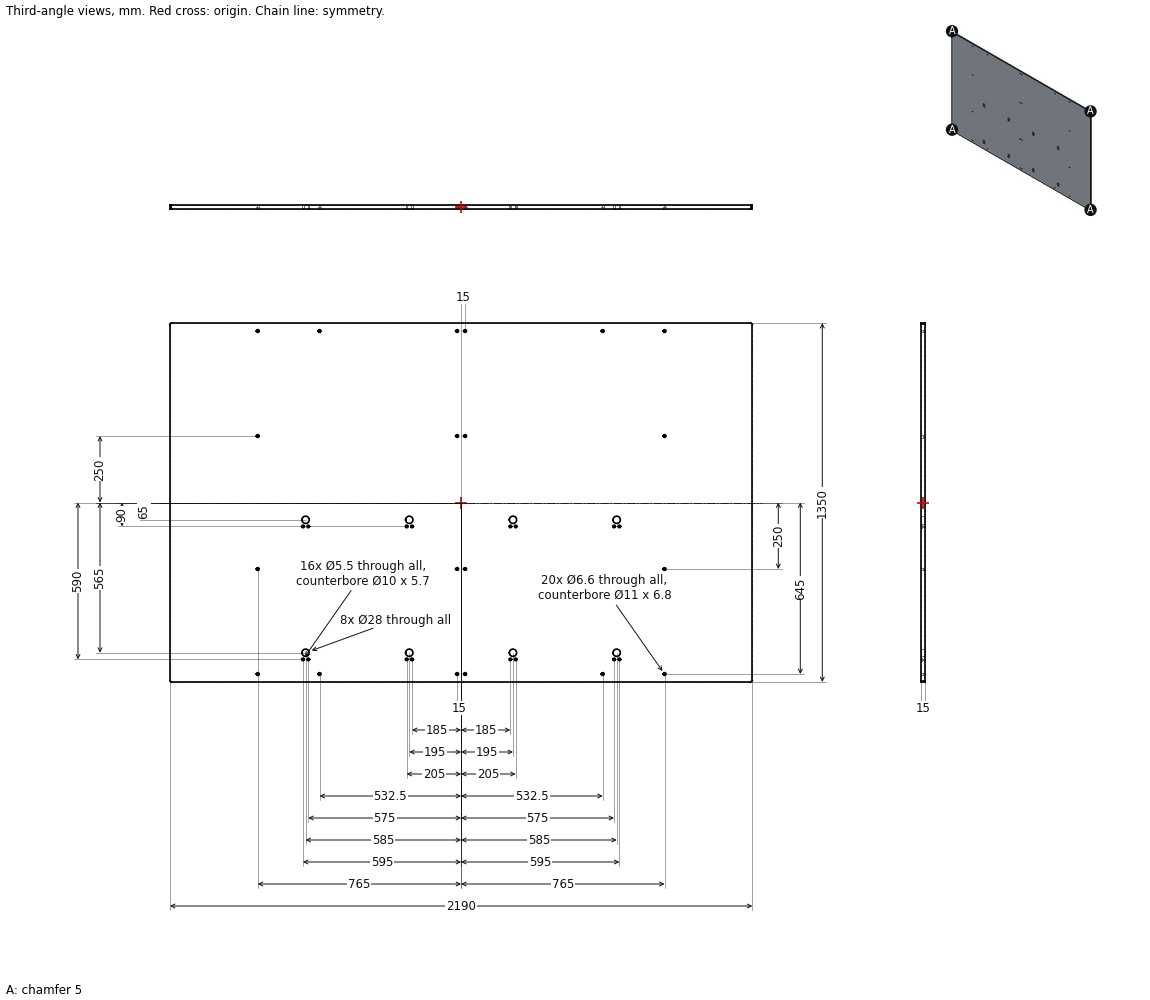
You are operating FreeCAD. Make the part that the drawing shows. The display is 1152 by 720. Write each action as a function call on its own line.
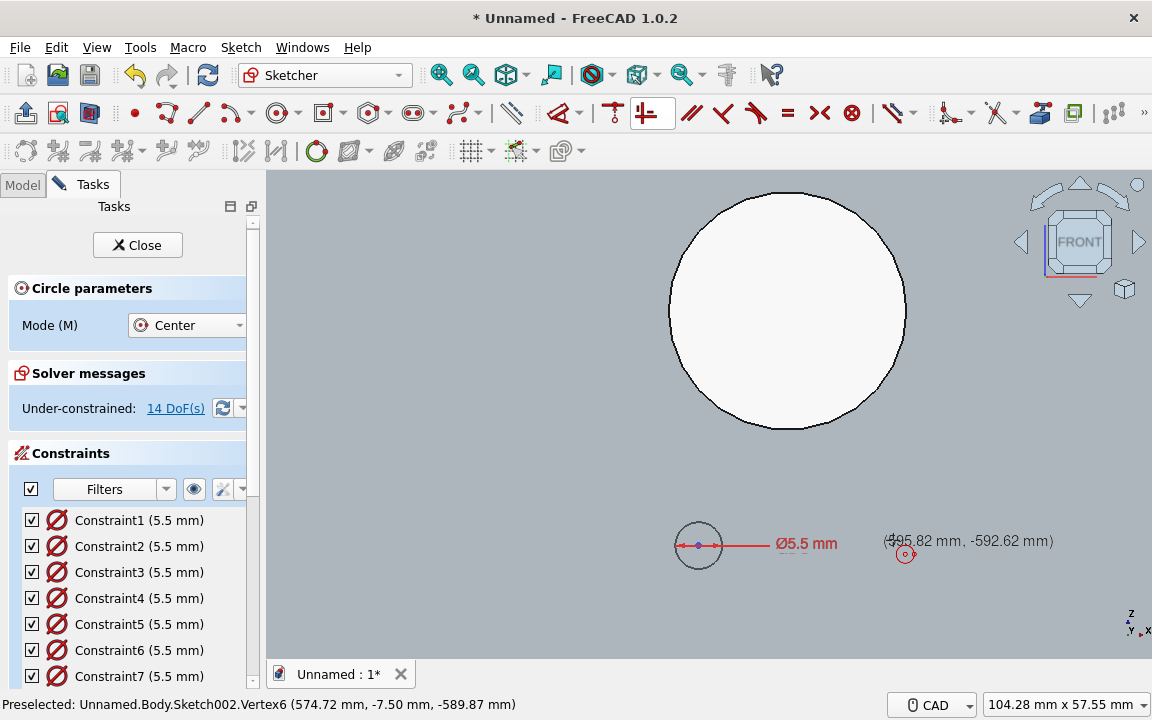
scroll(893, 540, down, 15)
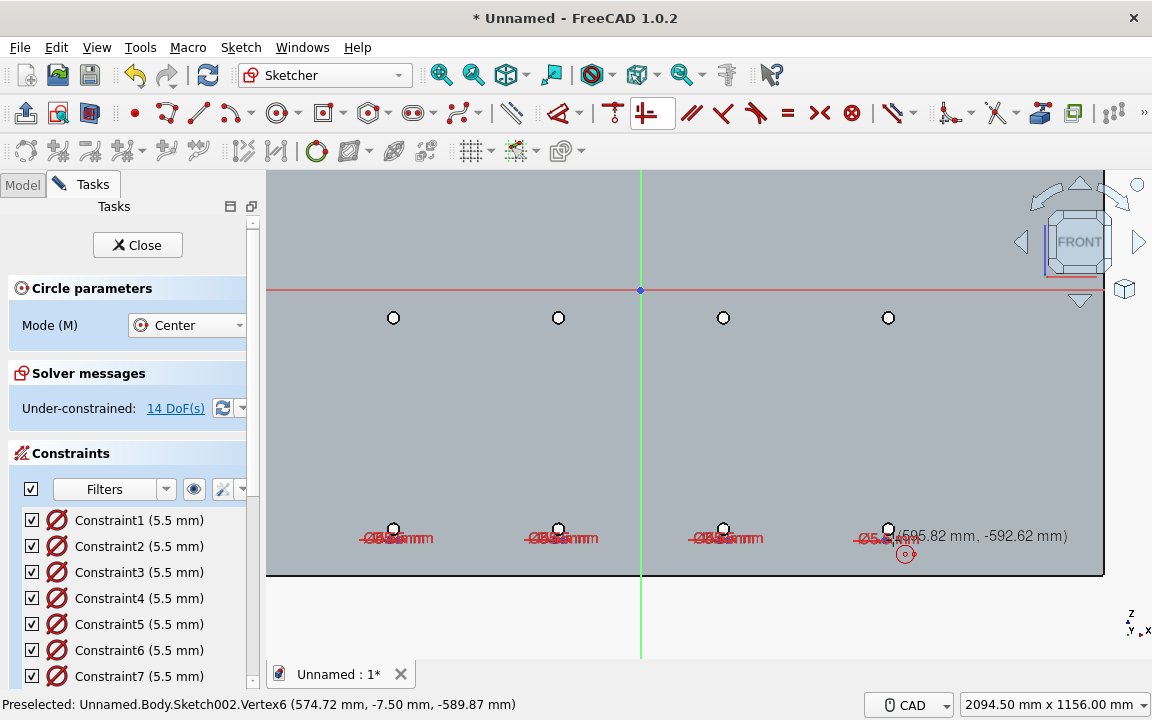
scroll(893, 540, up, 4)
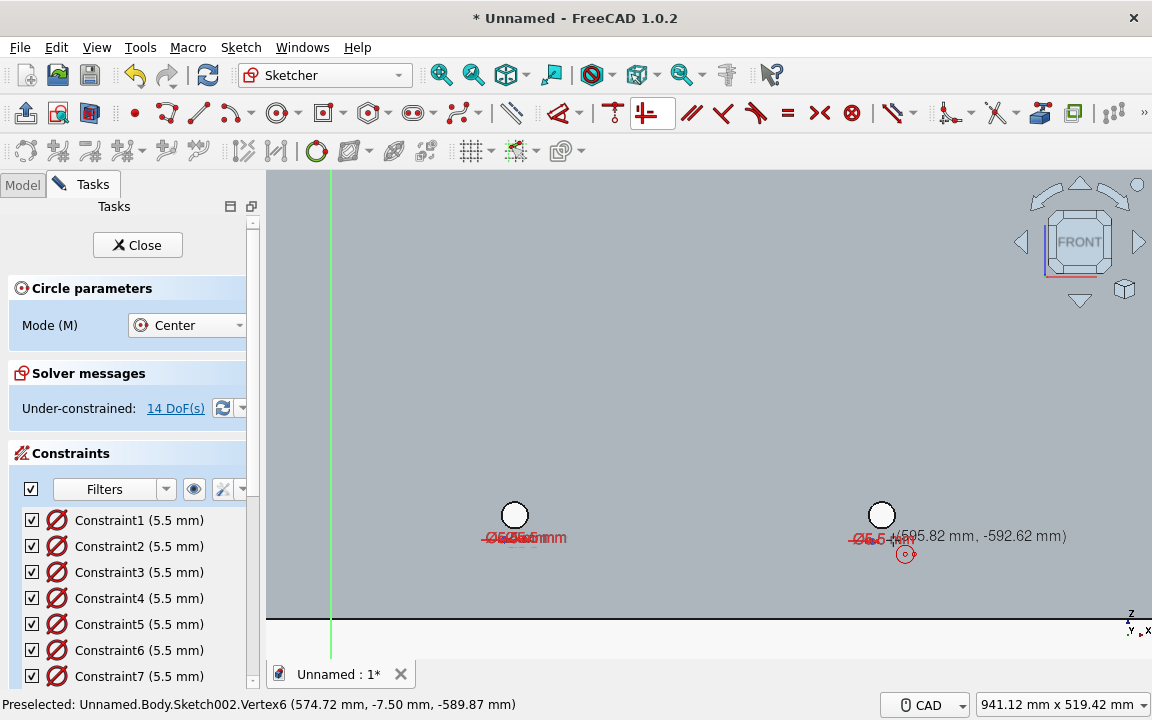
click(891, 539)
move(893, 537)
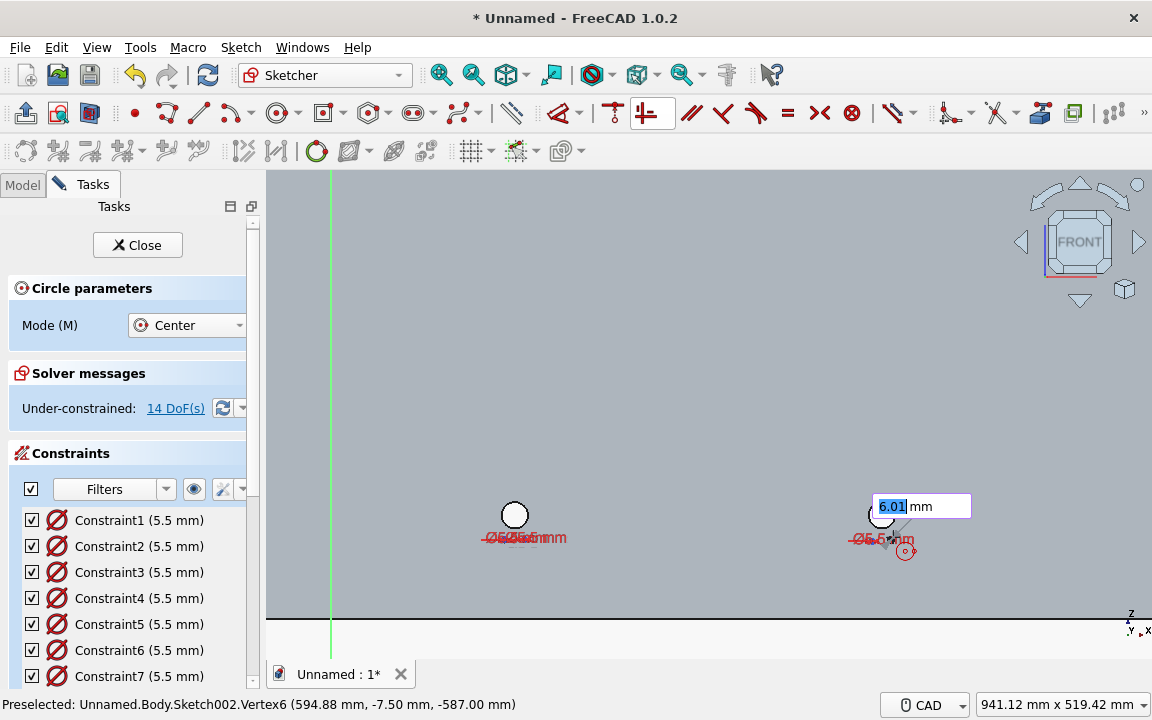
text(5.5)
key(Return)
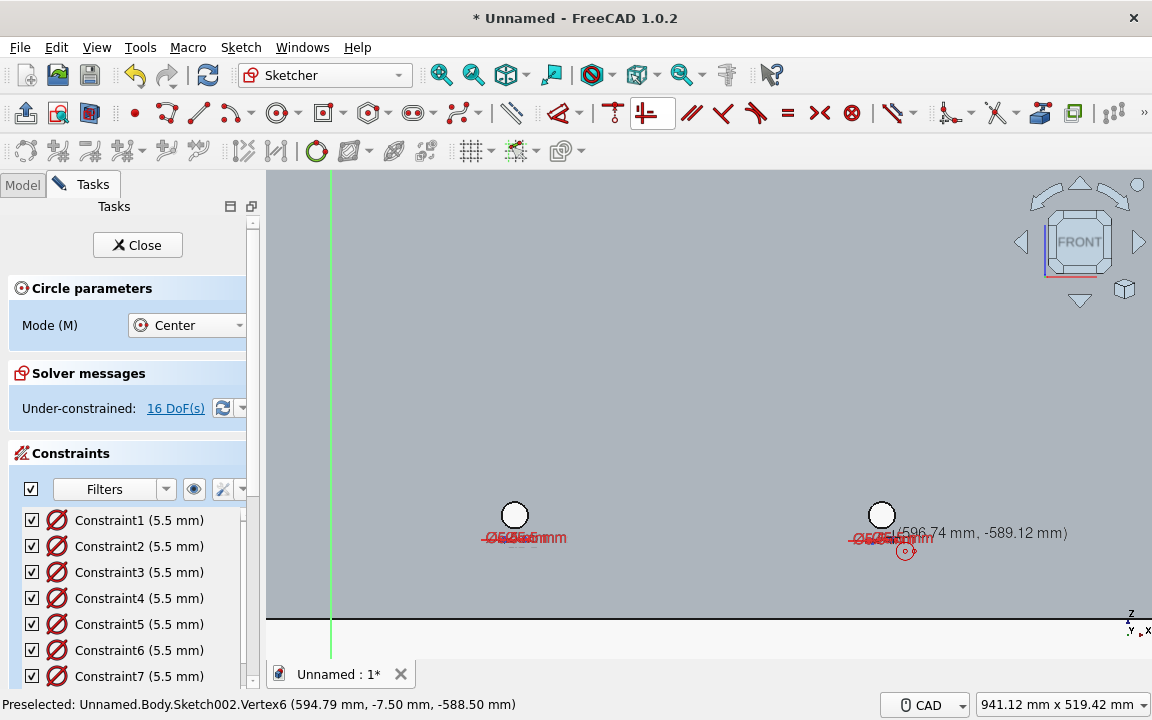
scroll(893, 539, down, 4)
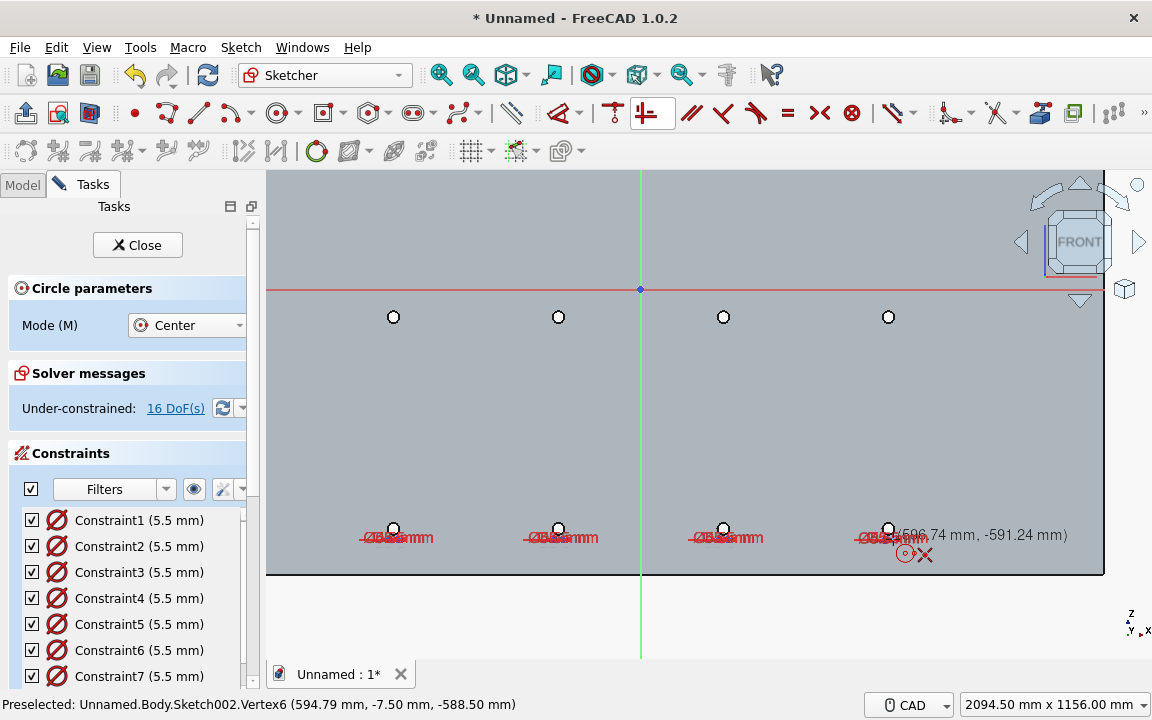
scroll(554, 328, up, 15)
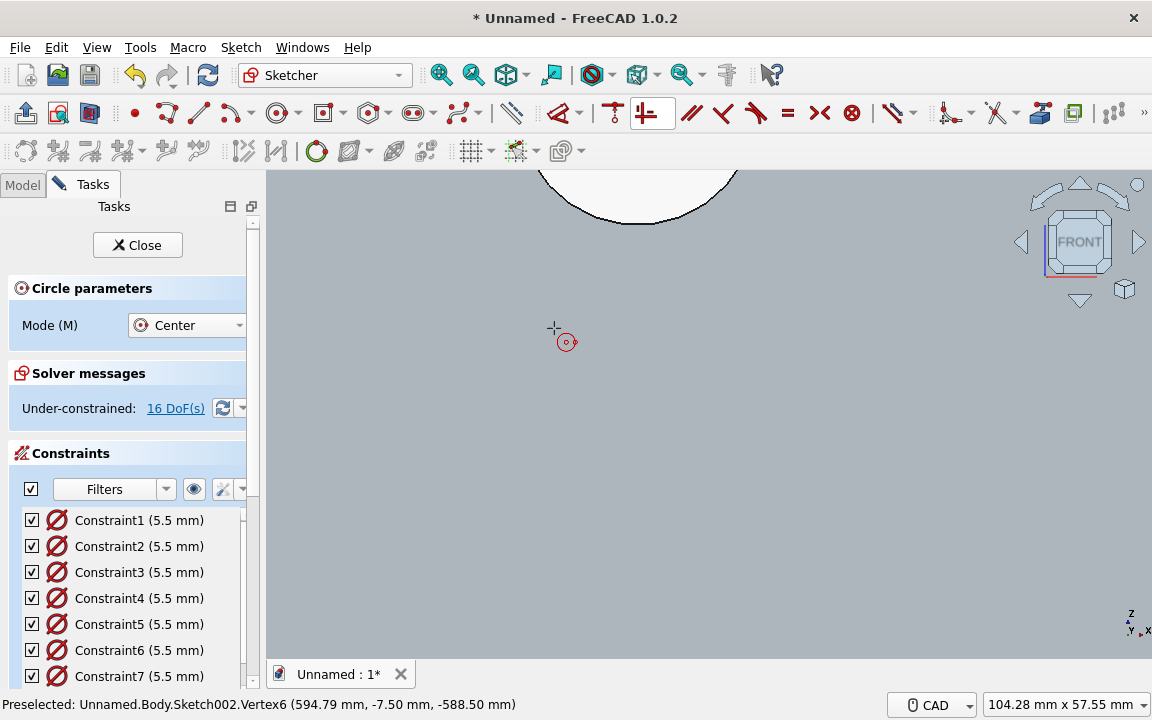
scroll(554, 328, down, 15)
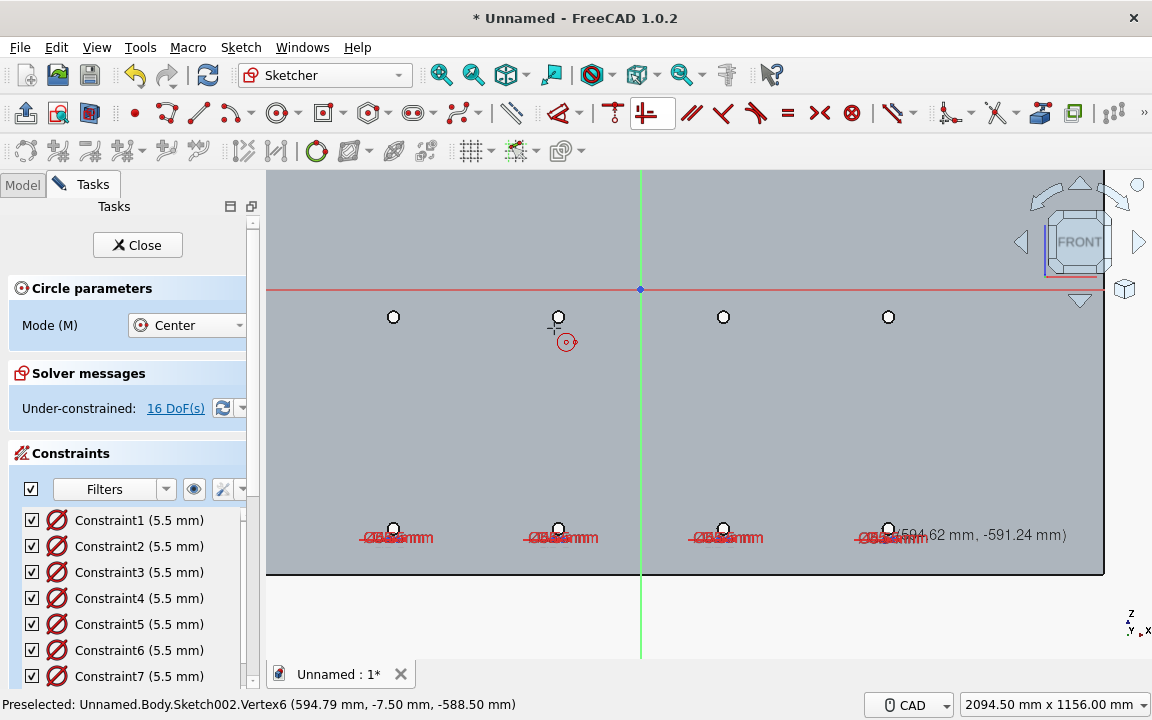
click(554, 328)
move(555, 327)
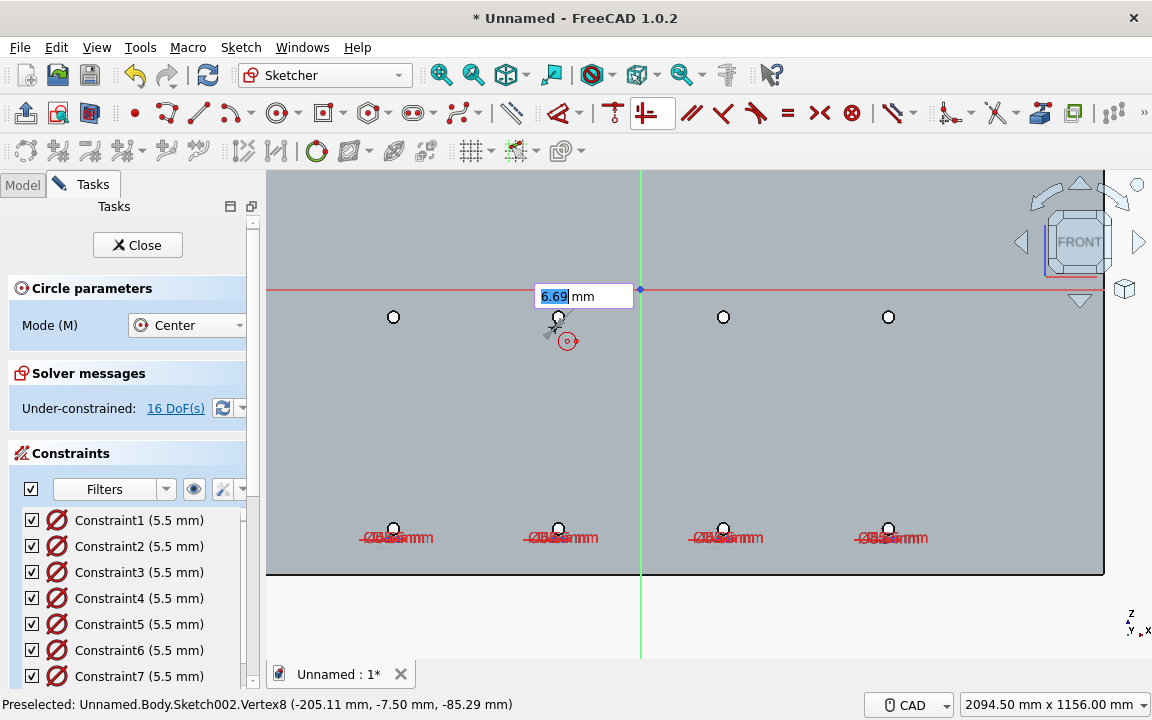
text(5.5)
key(Return)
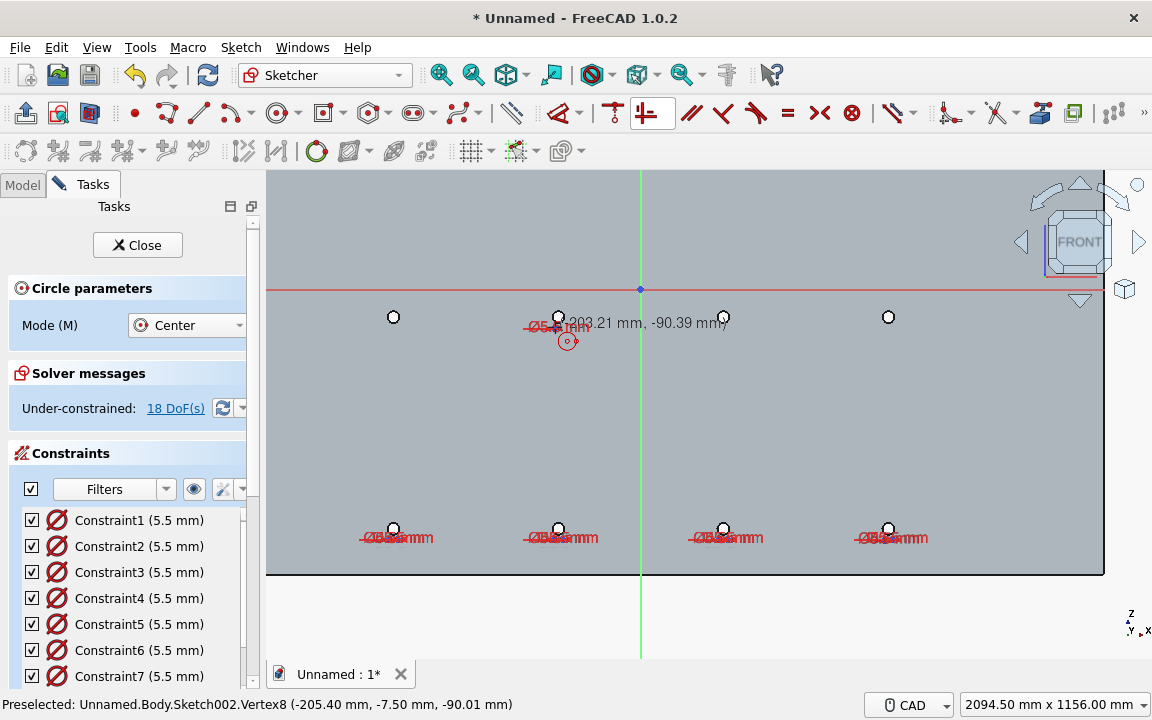
scroll(563, 328, up, 15)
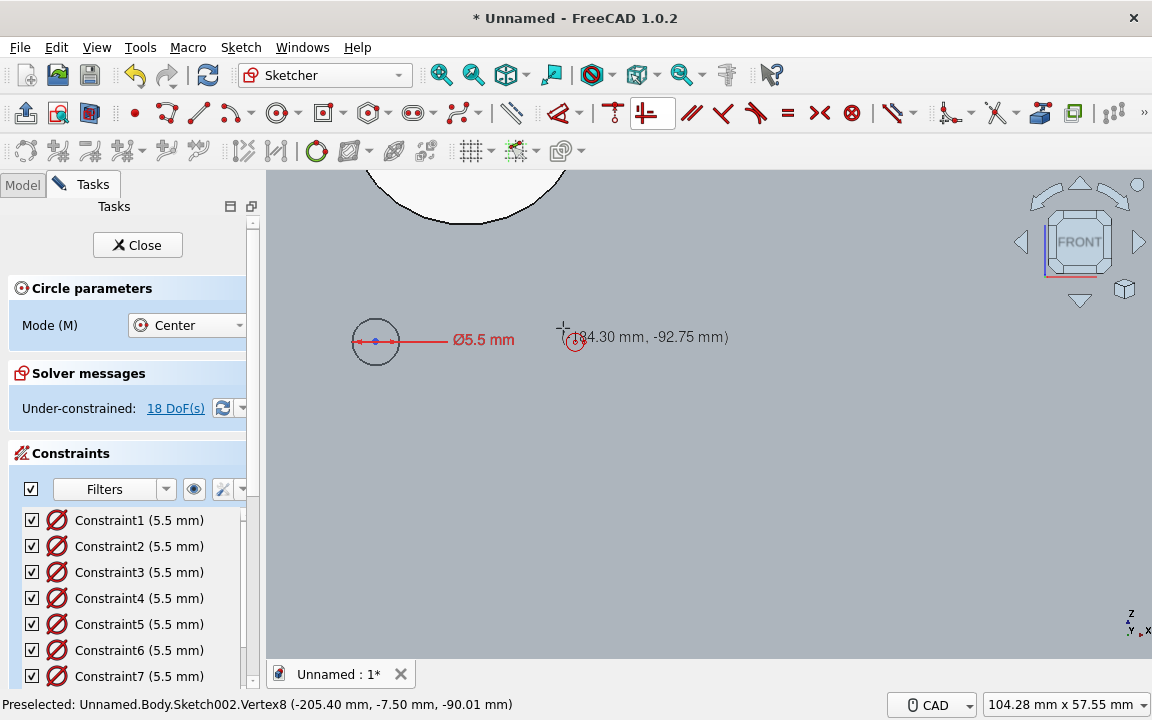
scroll(563, 328, down, 15)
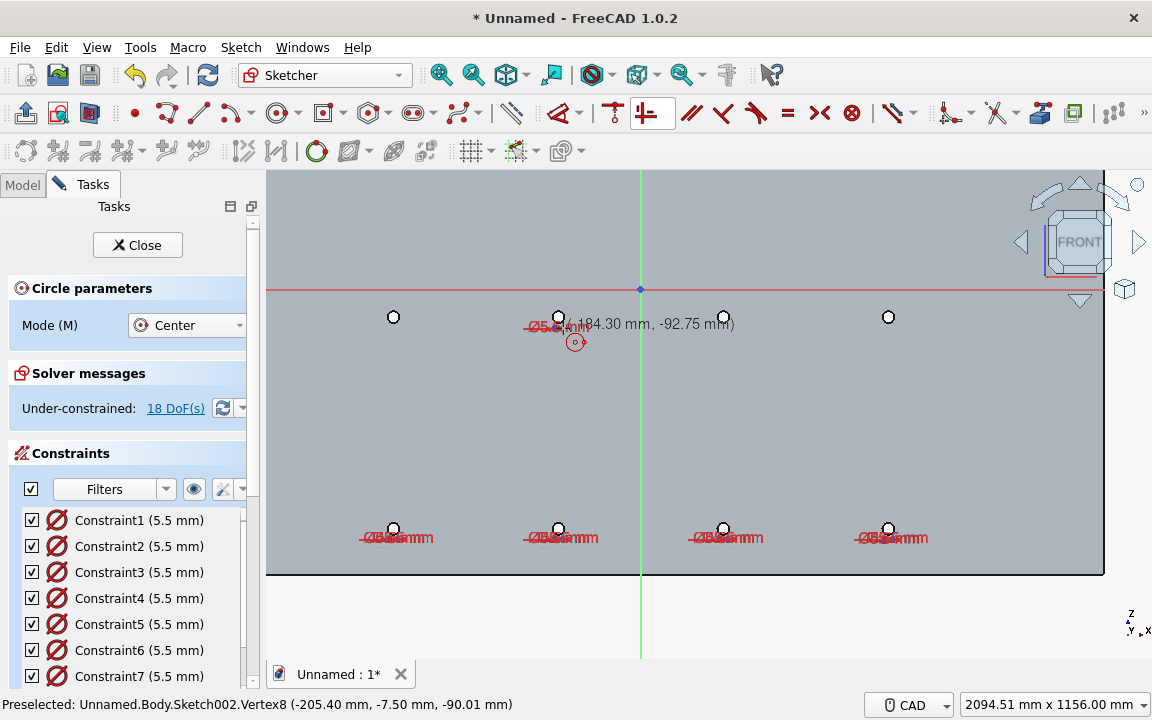
scroll(563, 328, up, 4)